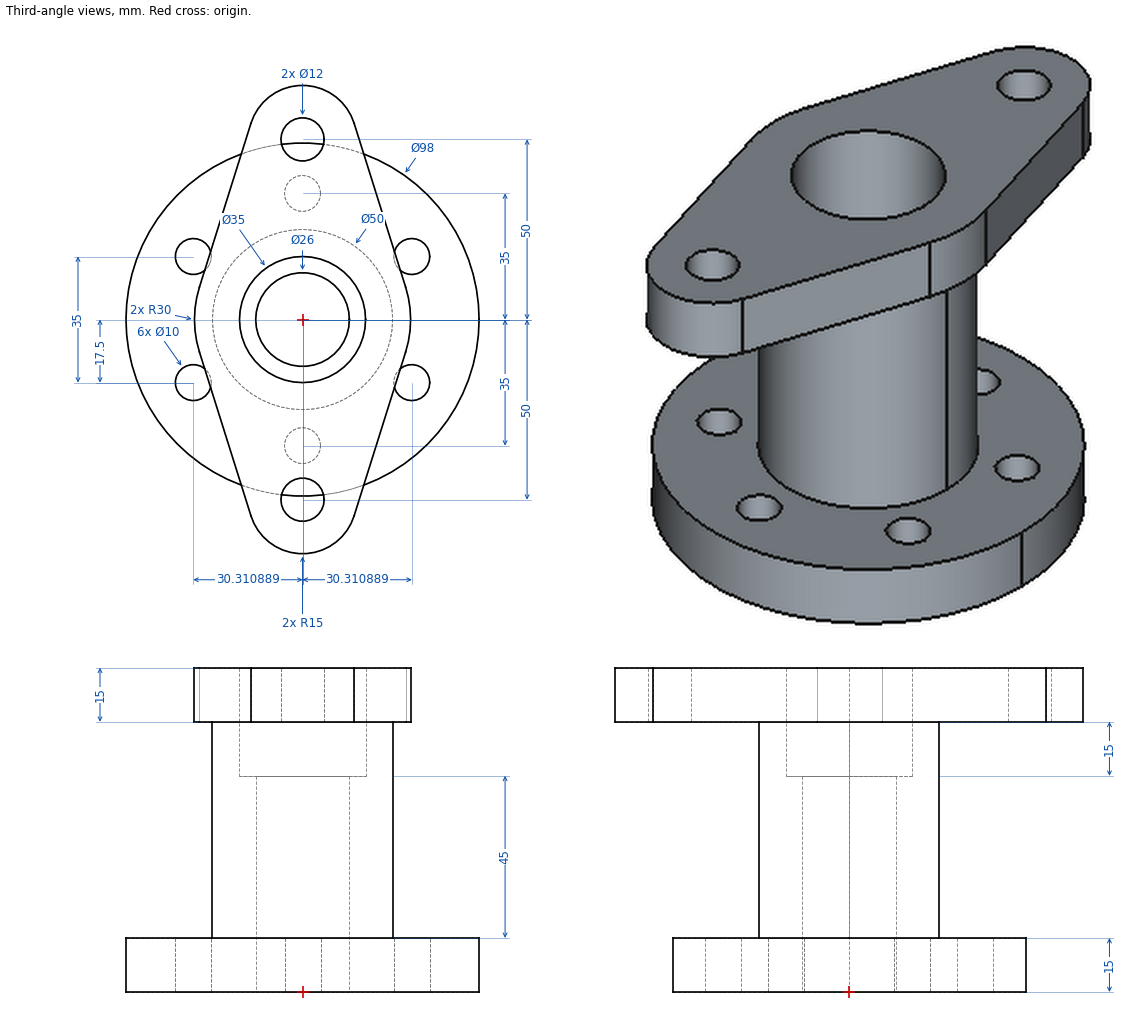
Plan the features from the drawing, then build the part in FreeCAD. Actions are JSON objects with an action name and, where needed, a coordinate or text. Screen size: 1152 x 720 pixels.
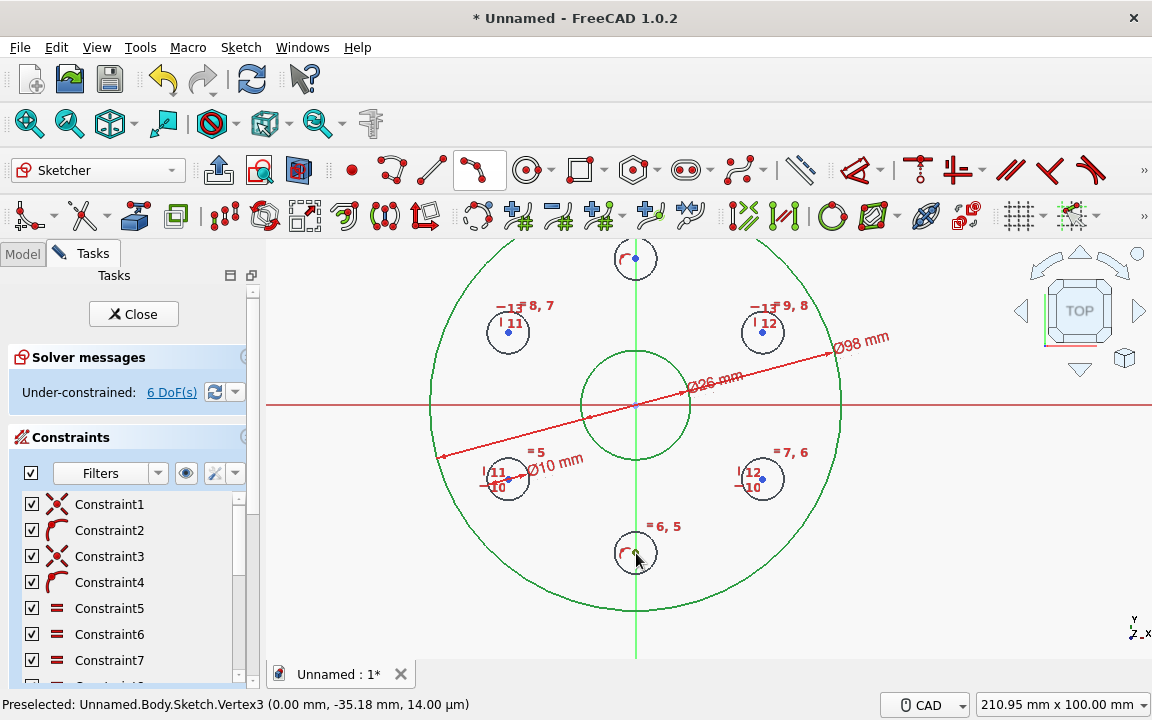
{"action": "key", "text": "i"}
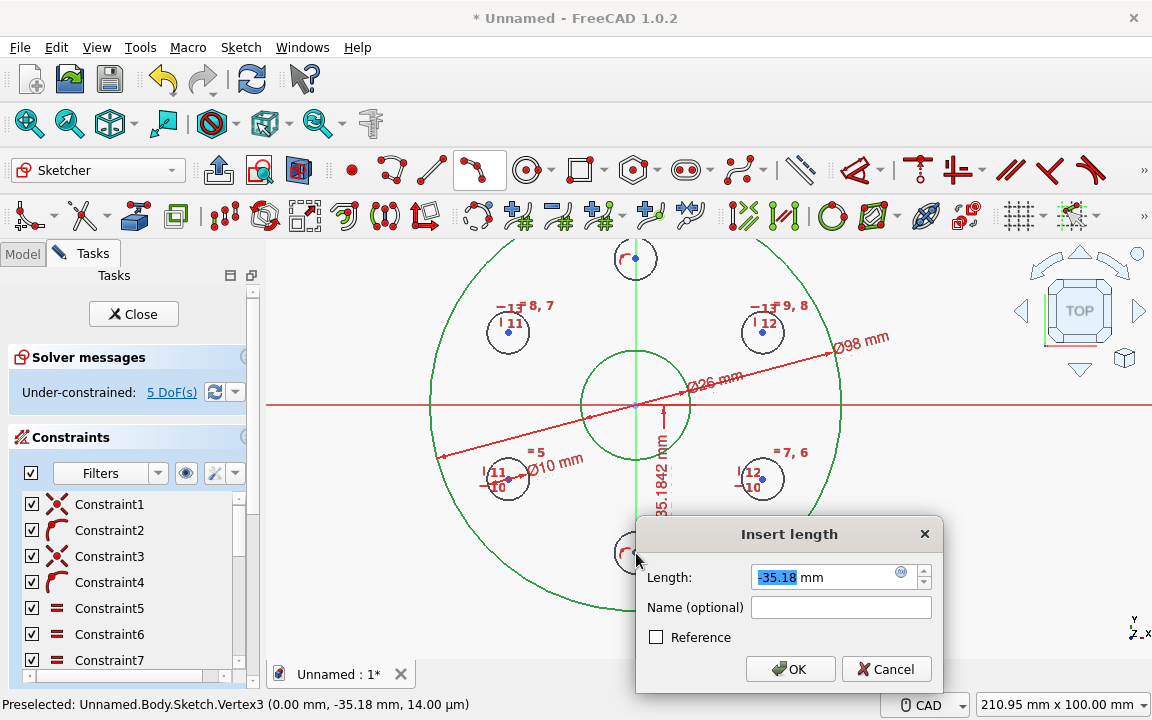
{"action": "type", "text": "-35"}
{"action": "key", "text": "Return"}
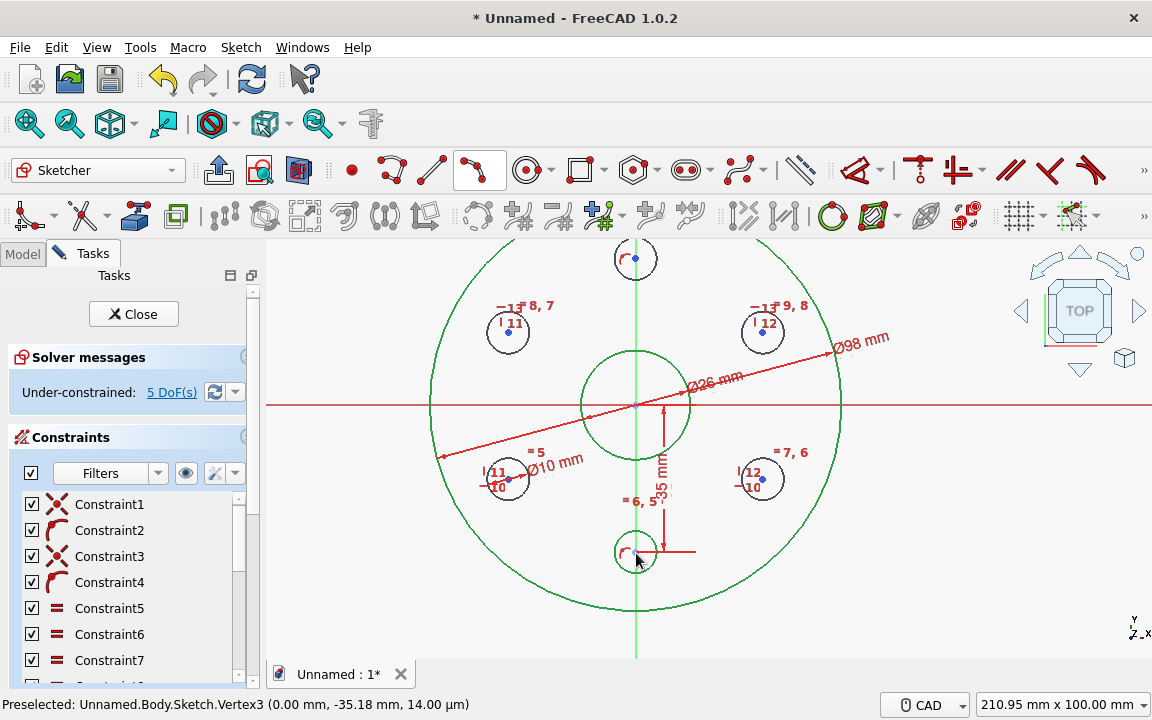
{"action": "scroll", "coordinate": [650, 538], "scroll_direction": "down", "scroll_amount": 2}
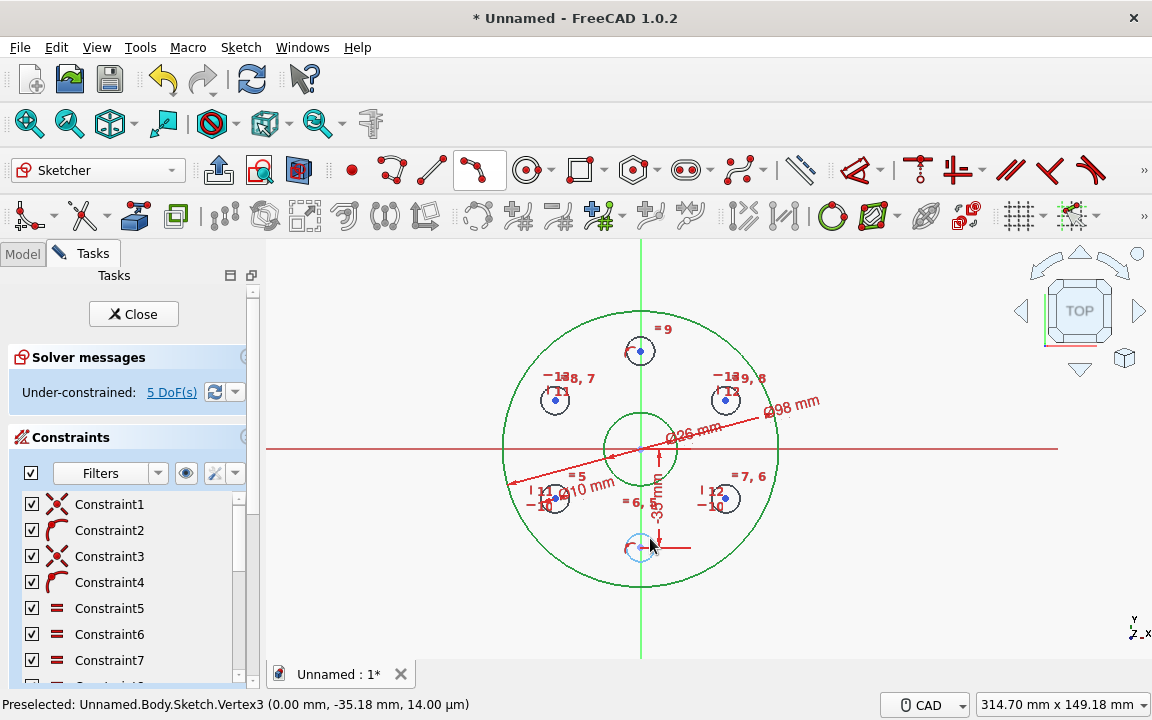
{"action": "left_click", "coordinate": [641, 351]}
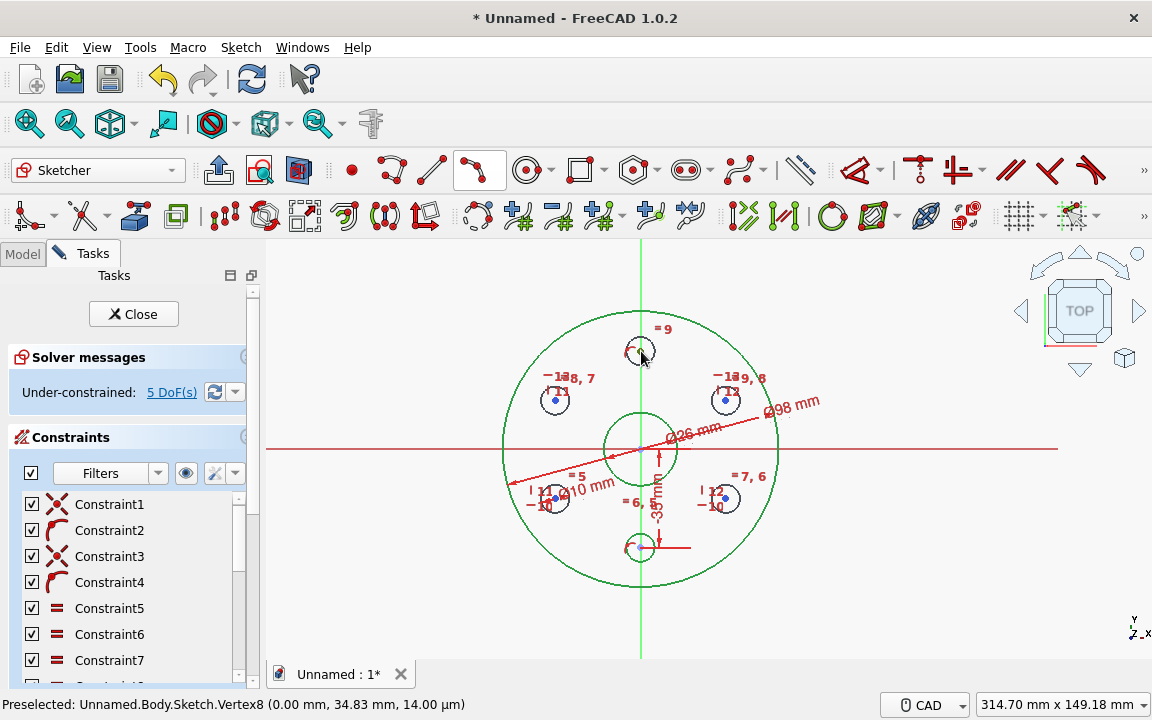
{"action": "key", "text": "i"}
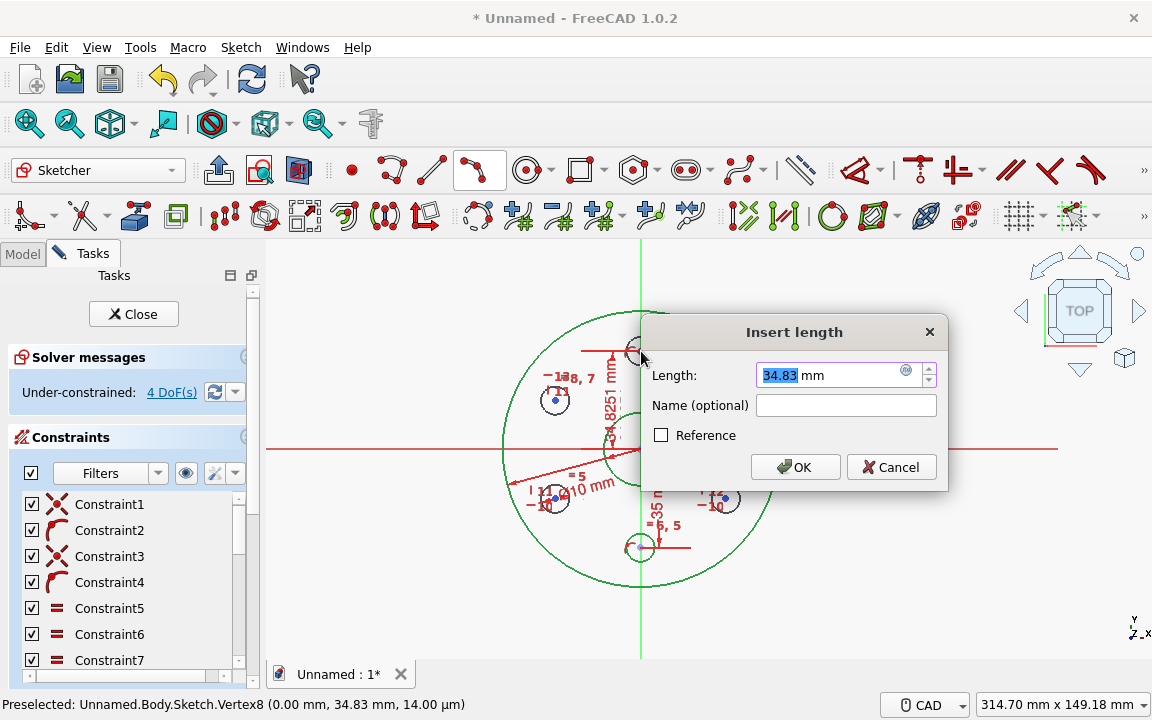
{"action": "type", "text": "35"}
{"action": "key", "text": "Return"}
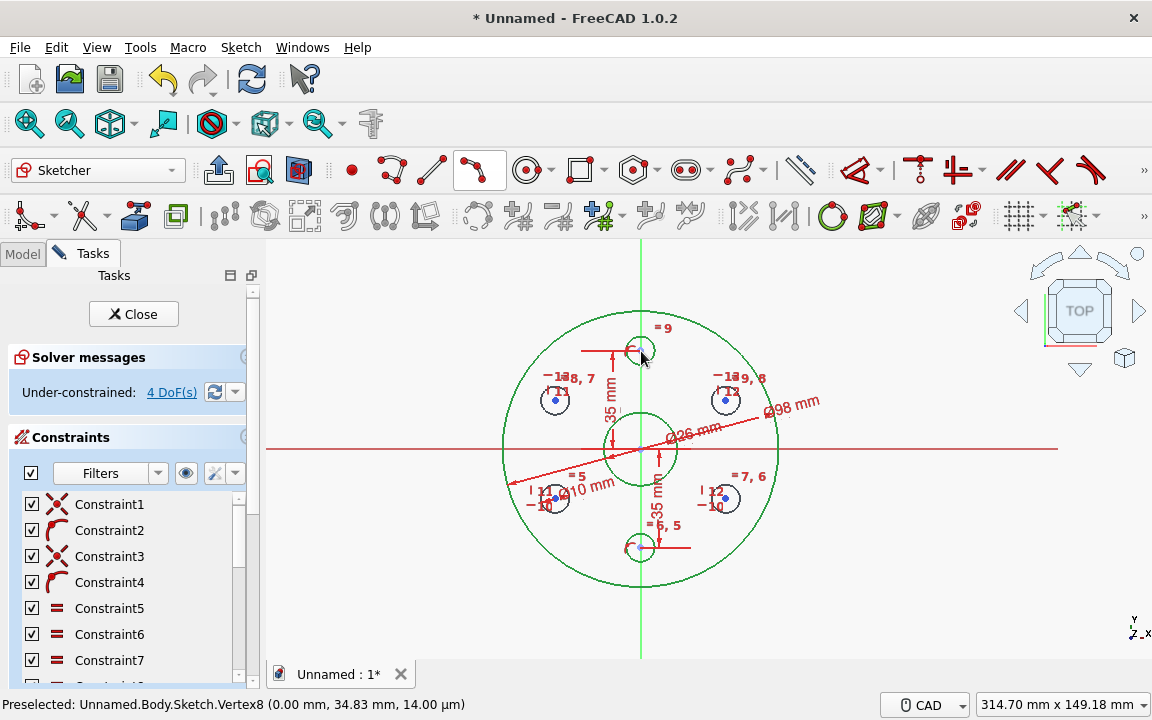
{"action": "left_click", "coordinate": [555, 499]}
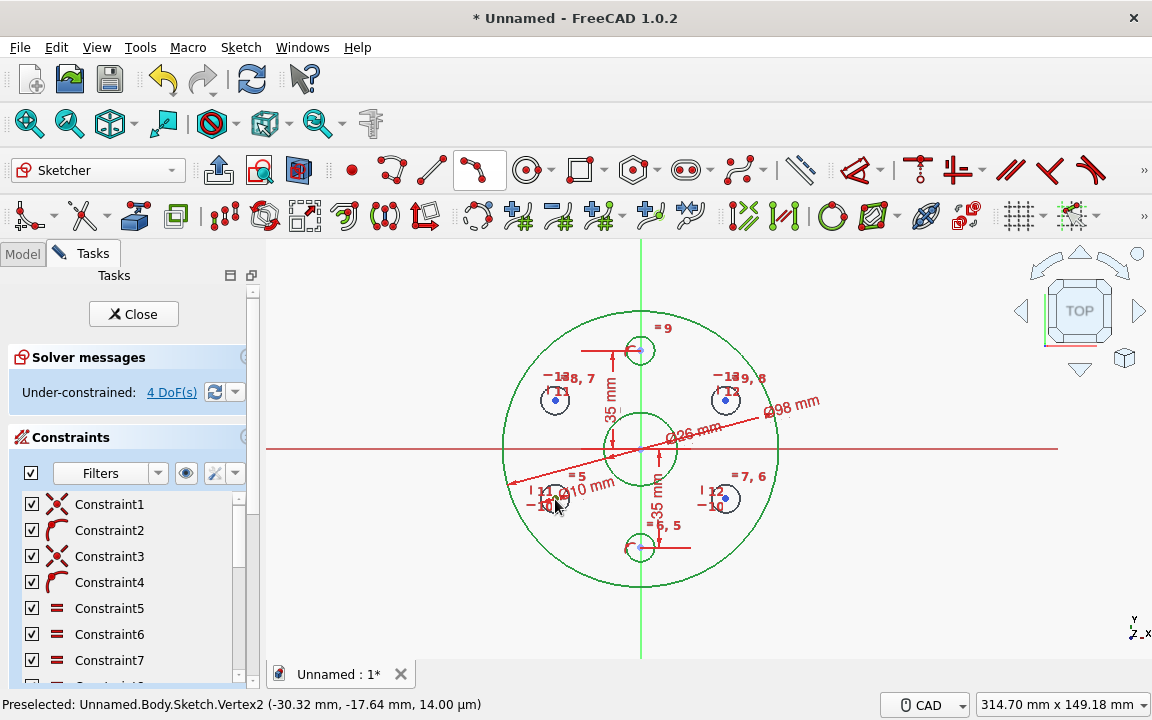
{"action": "left_click", "coordinate": [555, 401]}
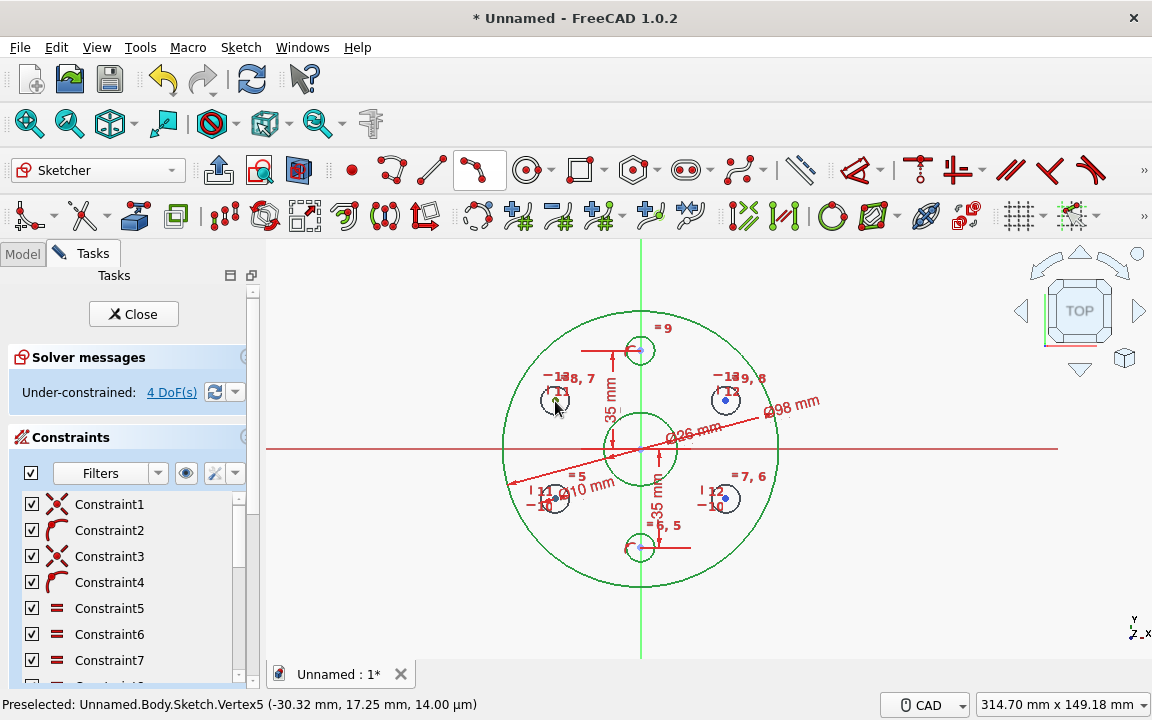
{"action": "key", "text": "i"}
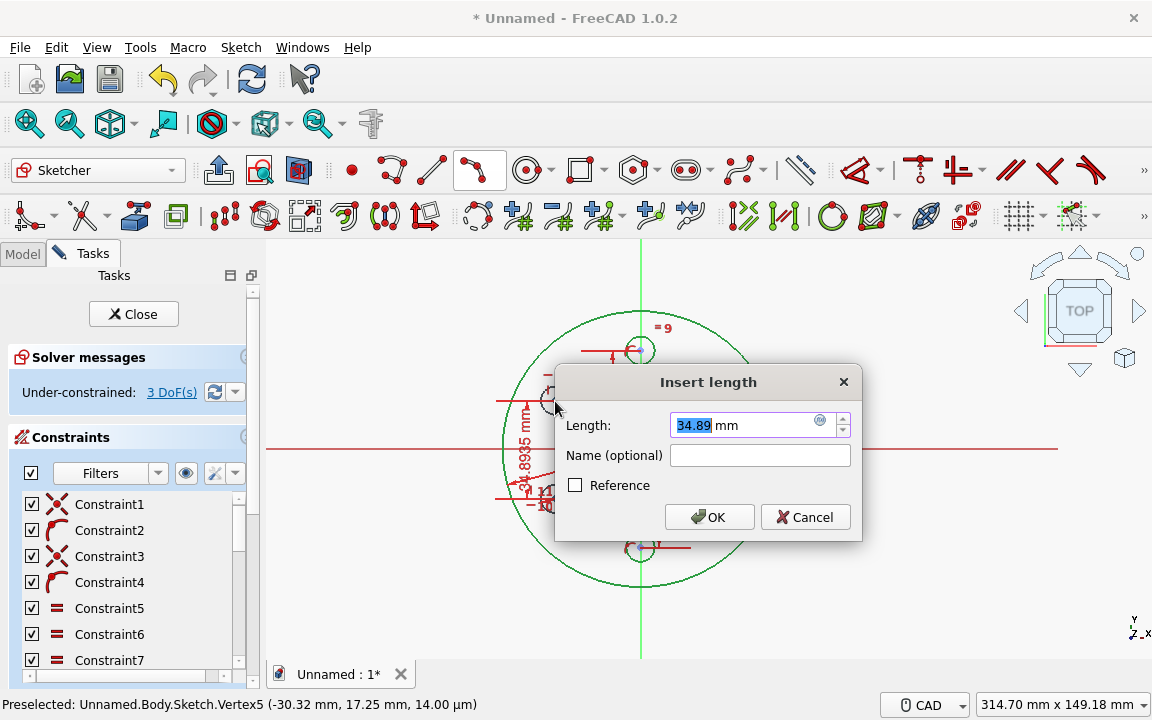
{"action": "type", "text": "35"}
{"action": "key", "text": "Return"}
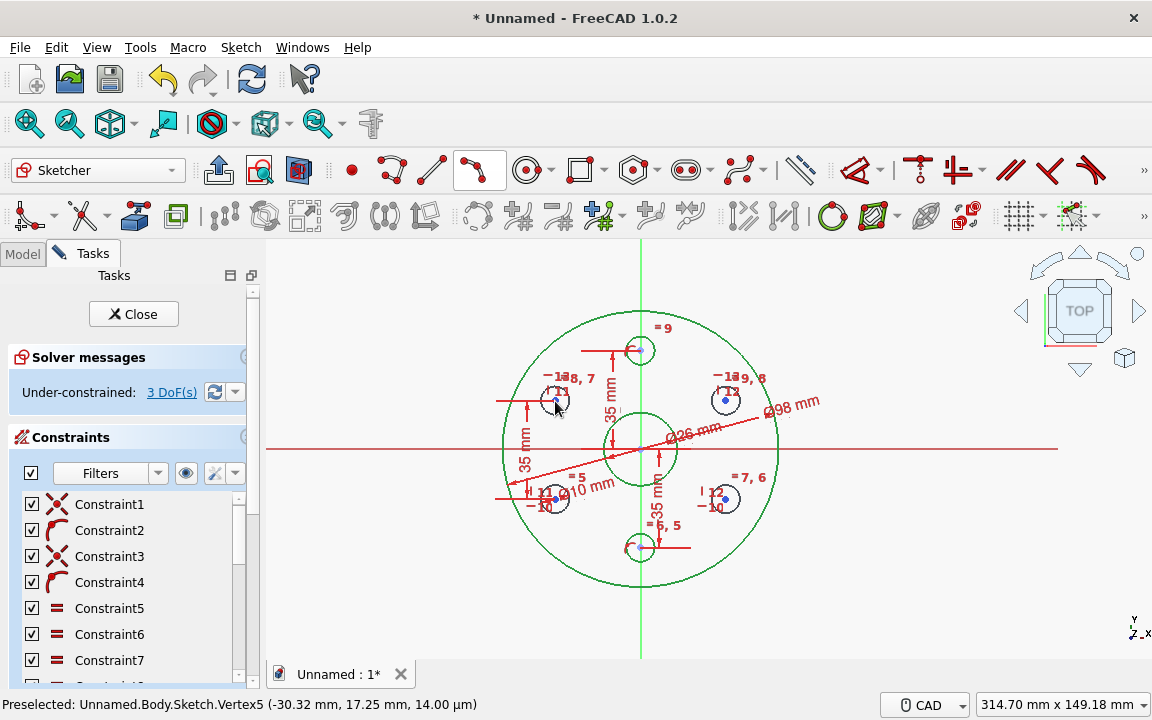
{"action": "left_click", "coordinate": [555, 499]}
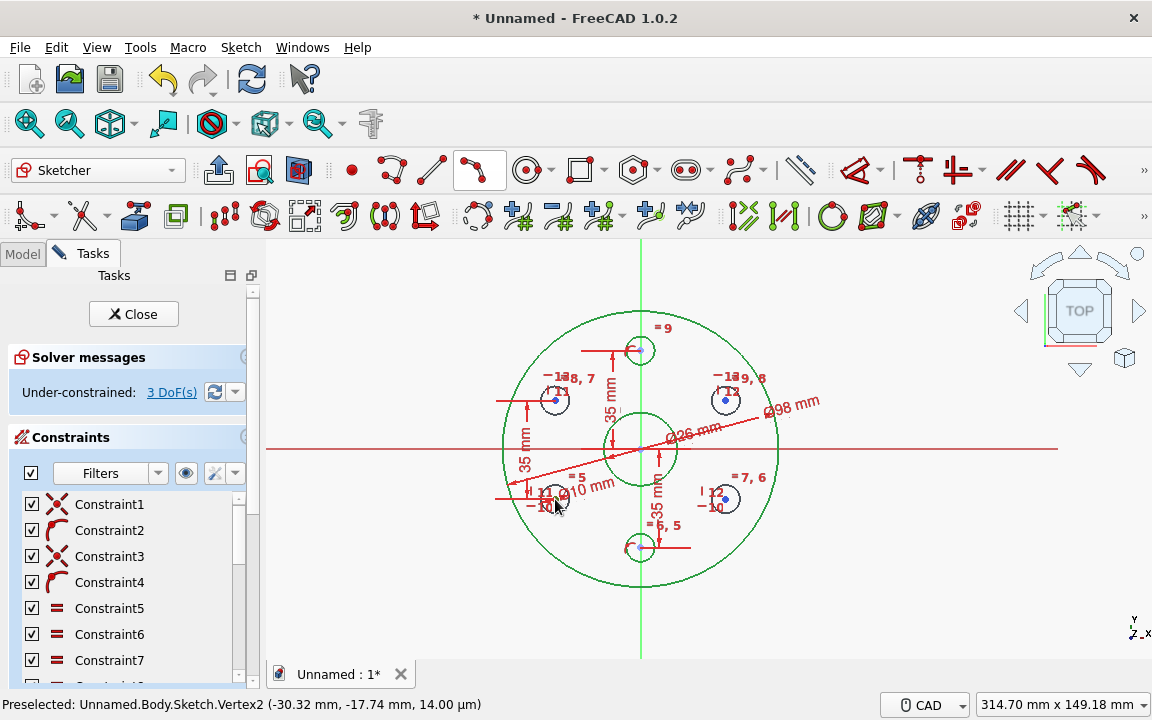
{"action": "key", "text": "i"}